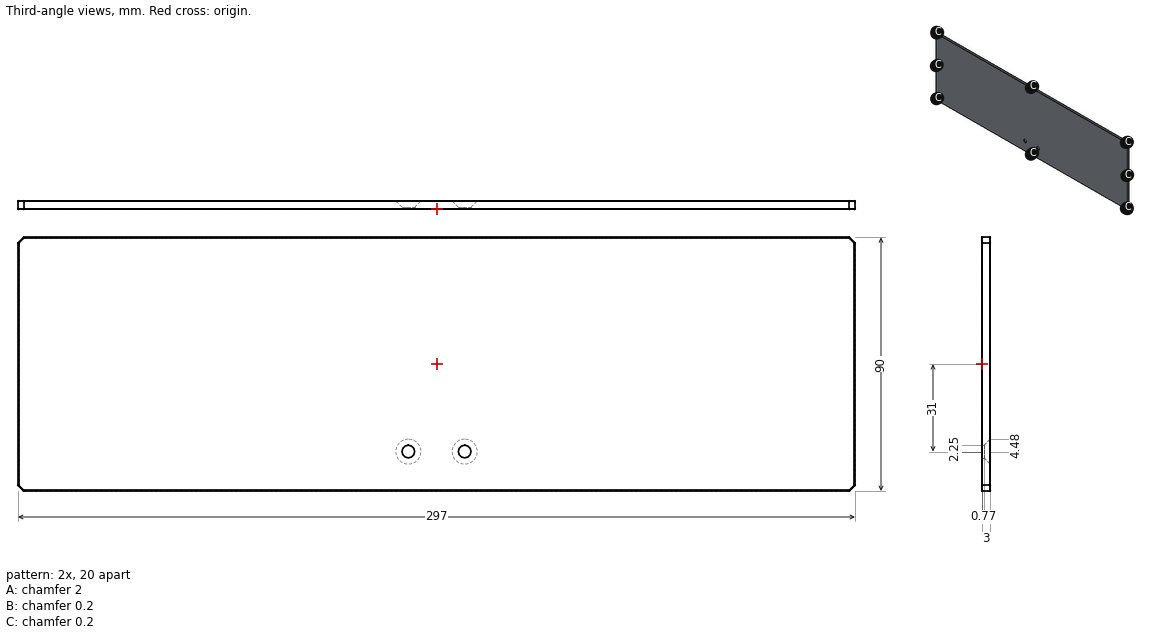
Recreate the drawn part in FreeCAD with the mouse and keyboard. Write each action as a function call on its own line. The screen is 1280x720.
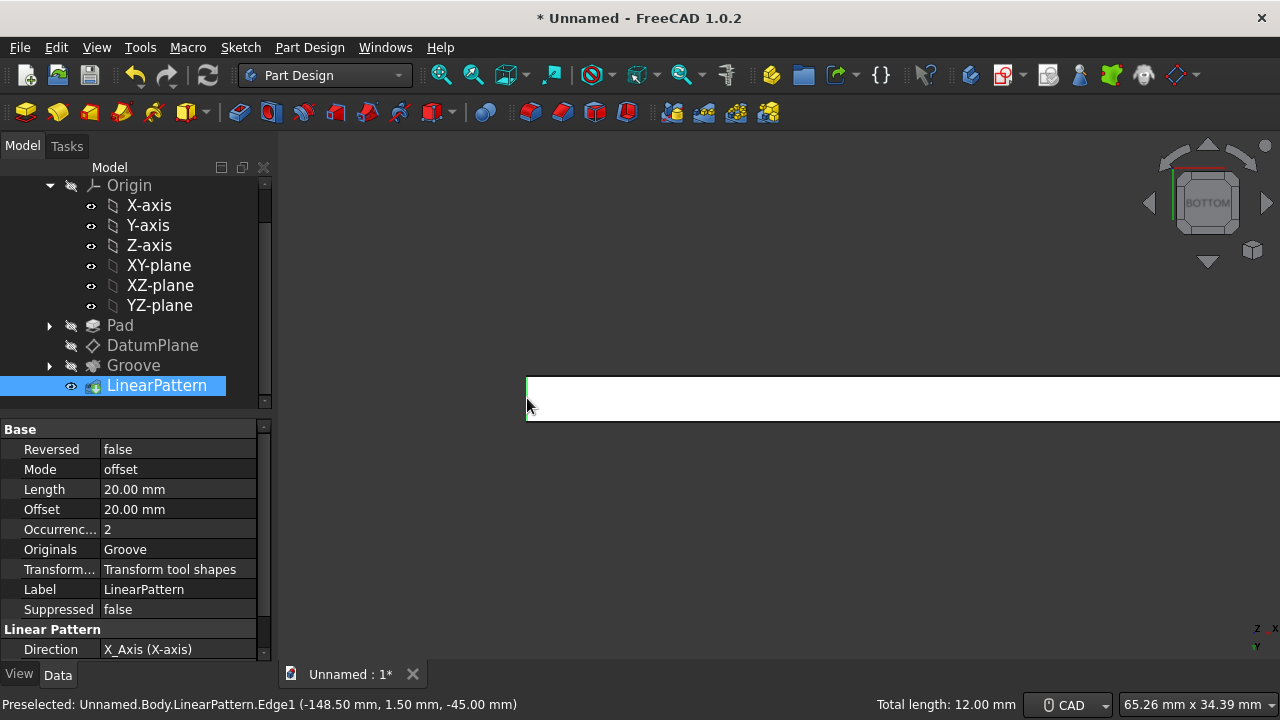
click(564, 112)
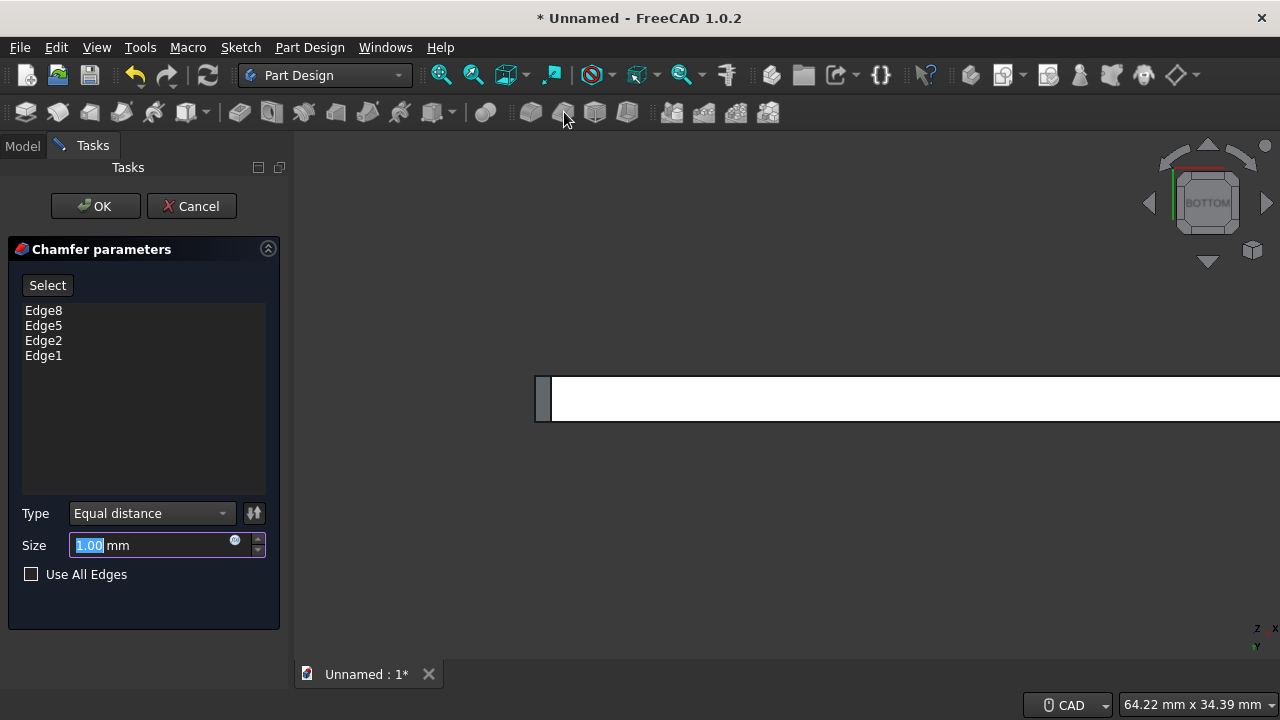
text(2)
key(Tab)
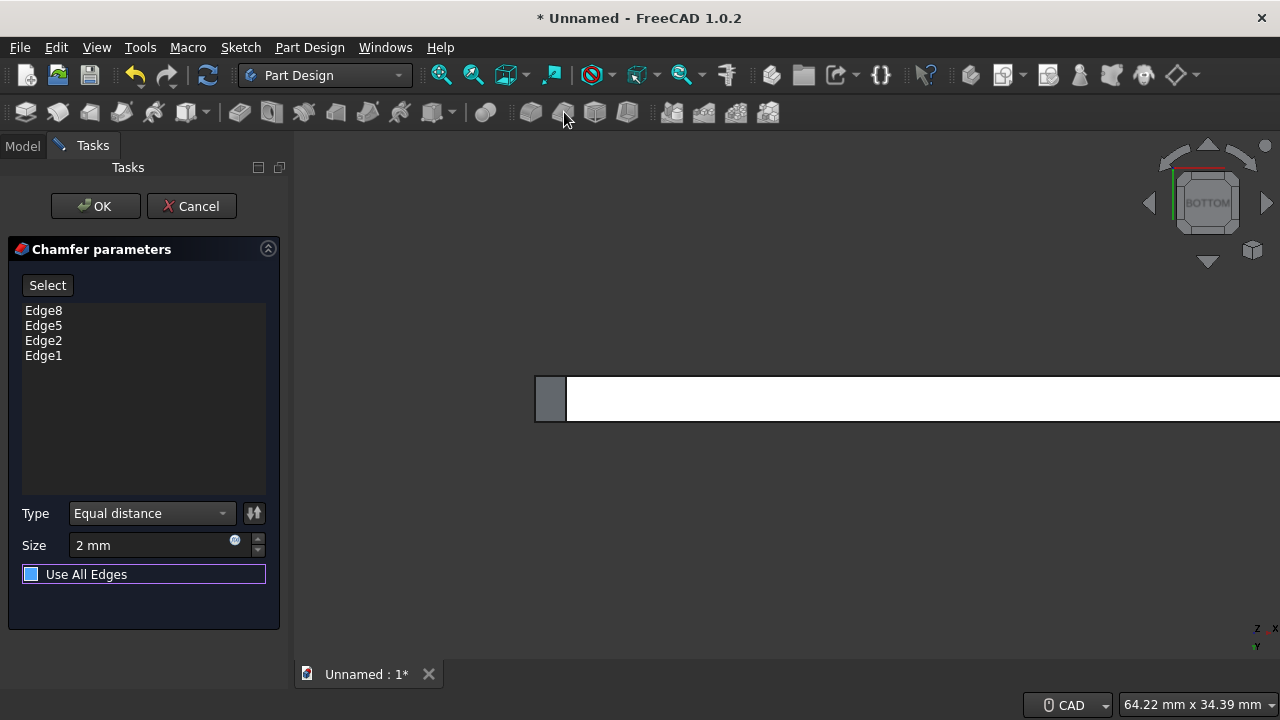
click(96, 206)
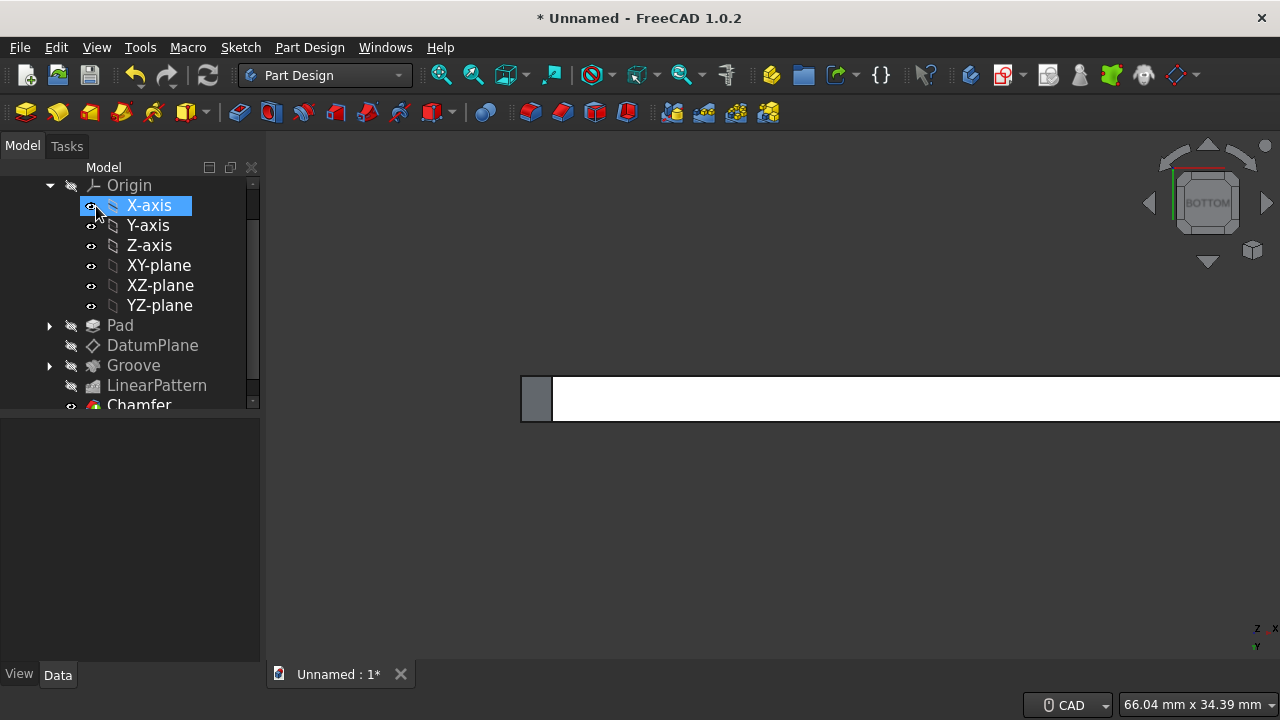
click(442, 76)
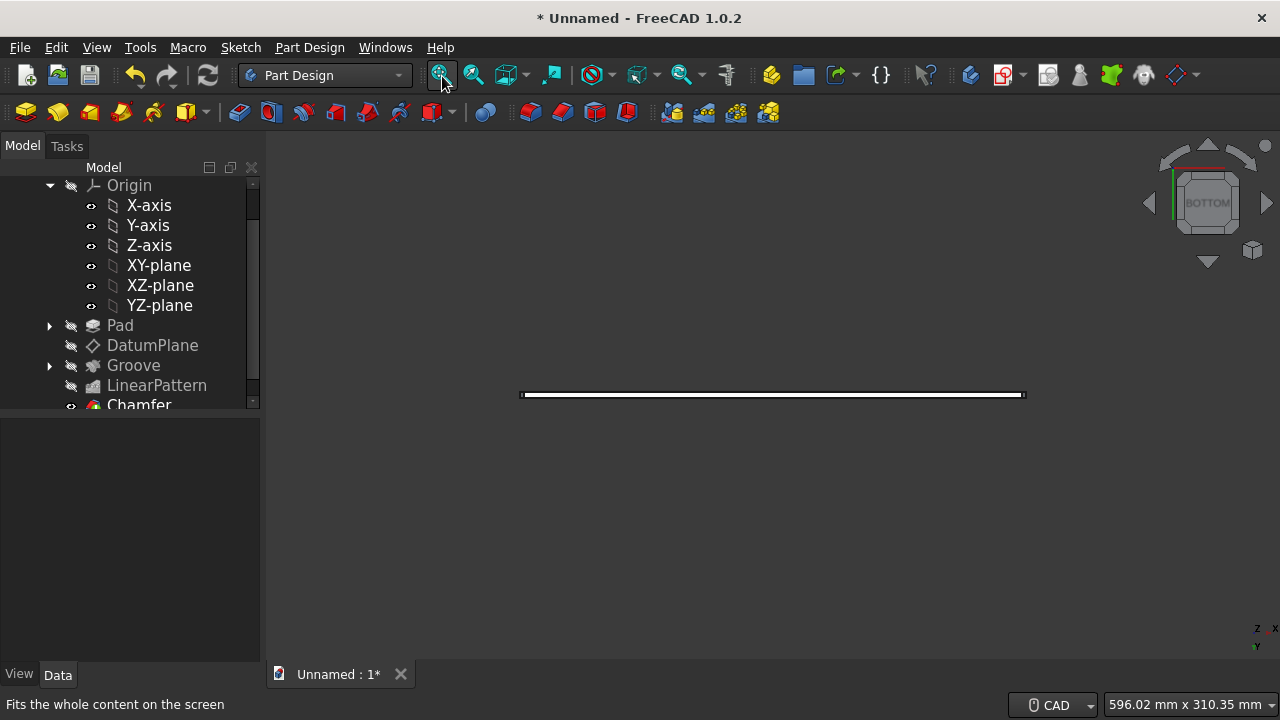
click(773, 391)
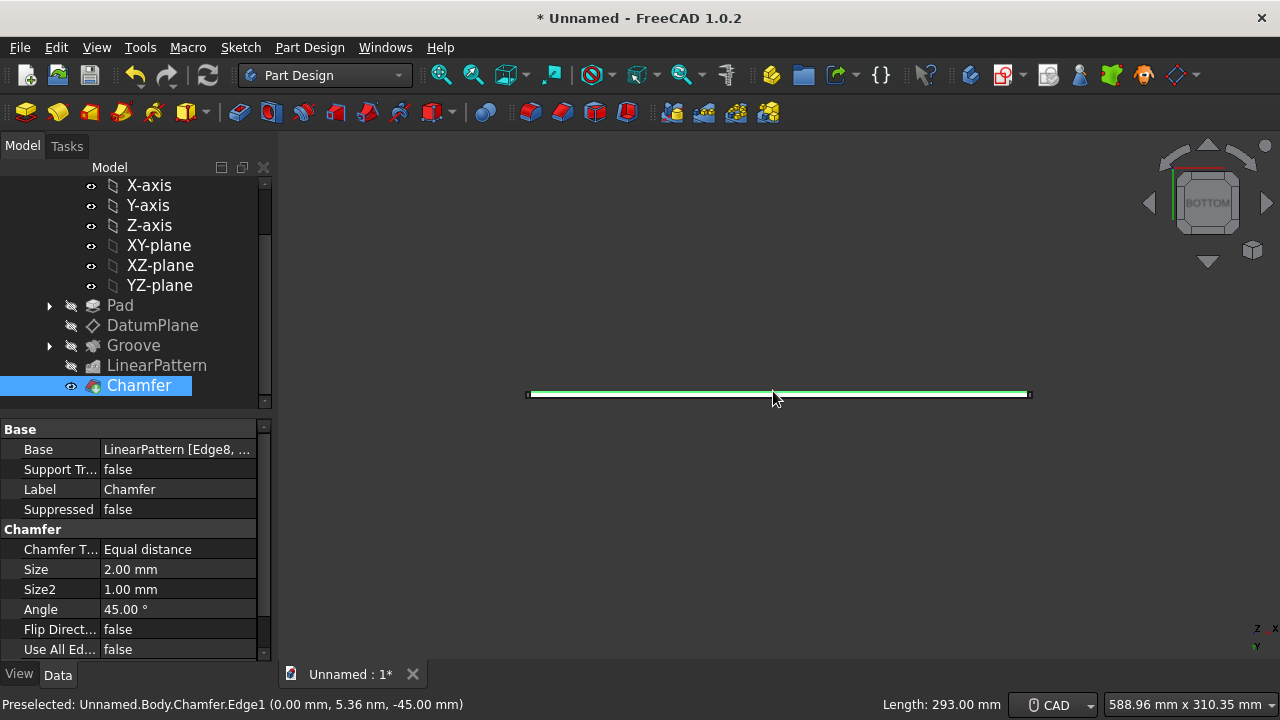
key(0)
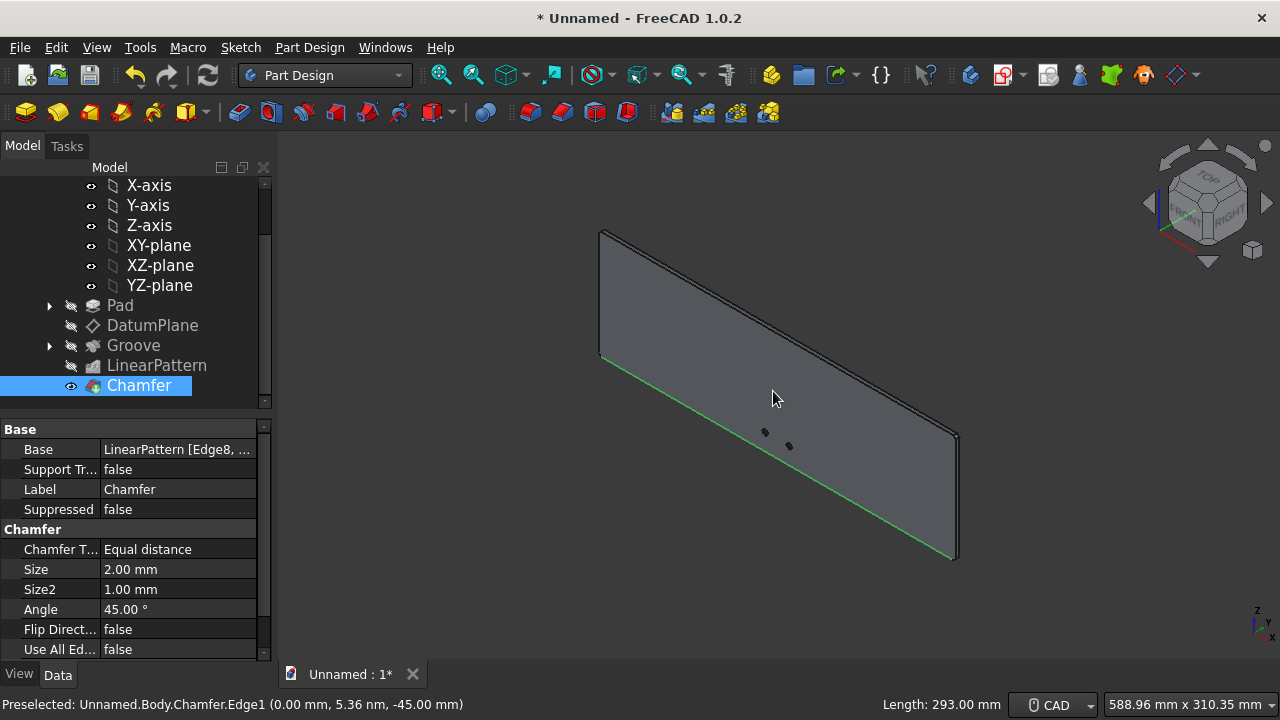
click(956, 498, ctrl)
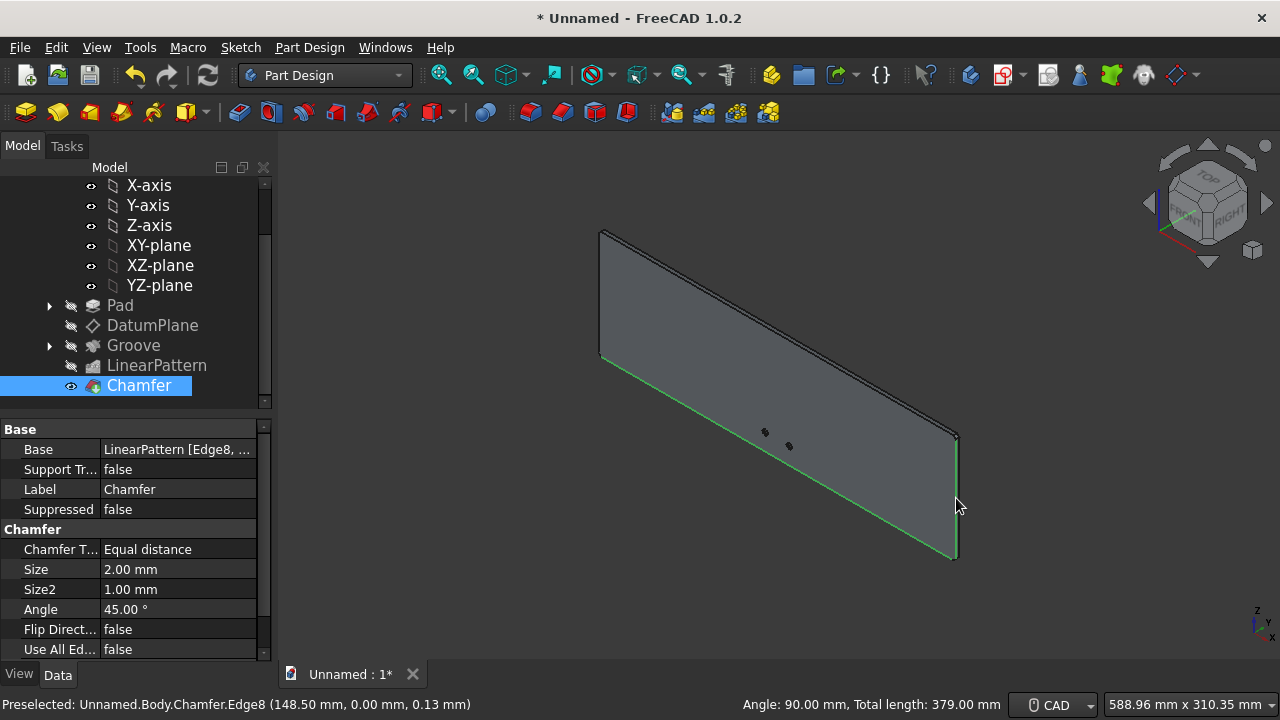
click(777, 333, ctrl)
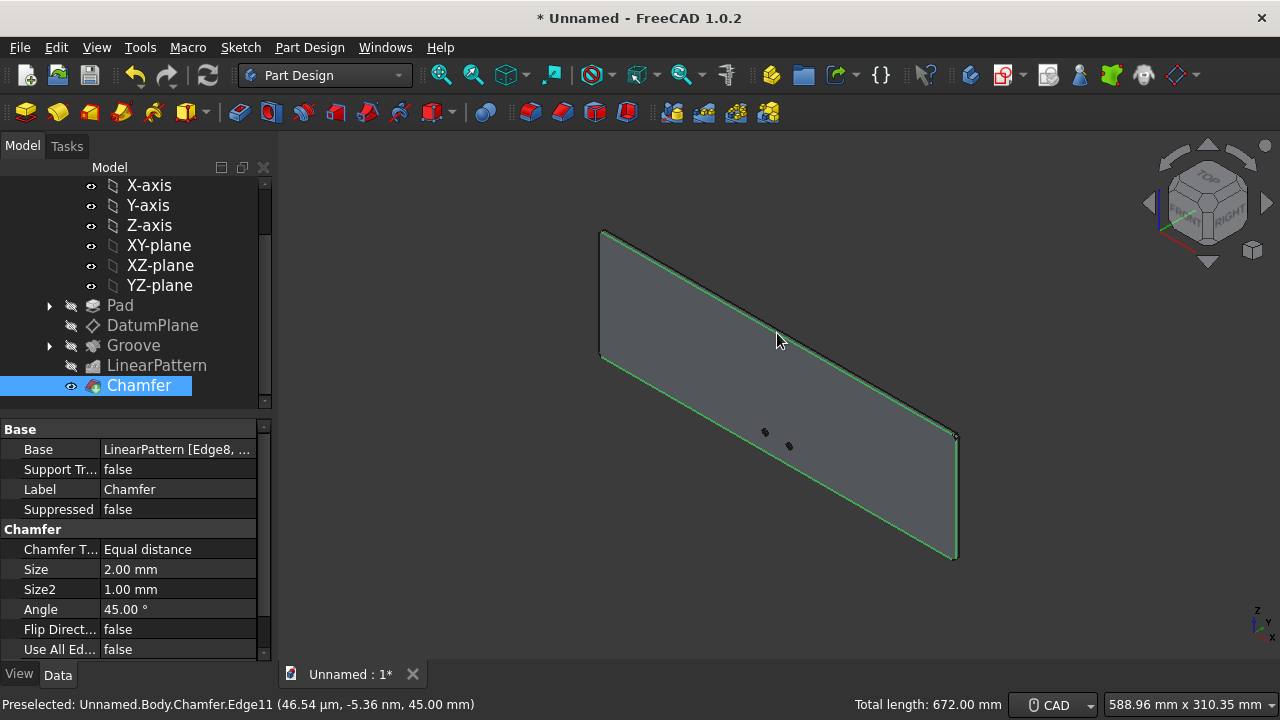
key(2)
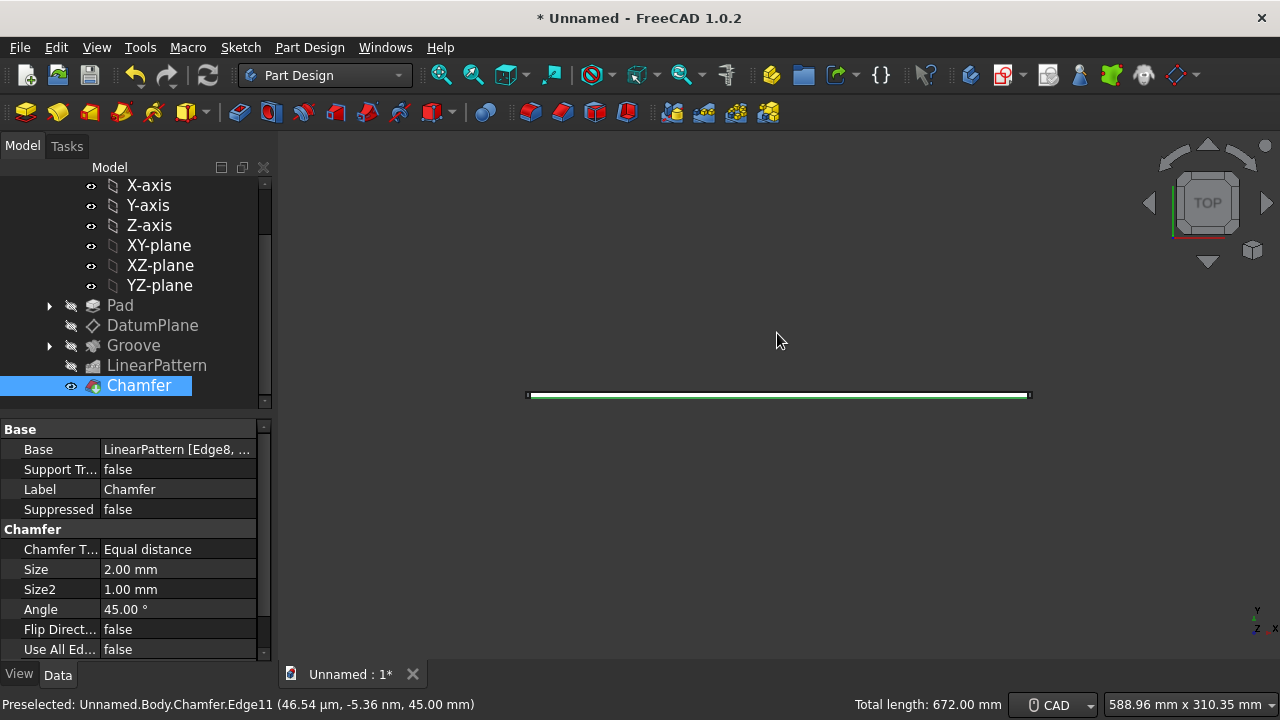
key(1)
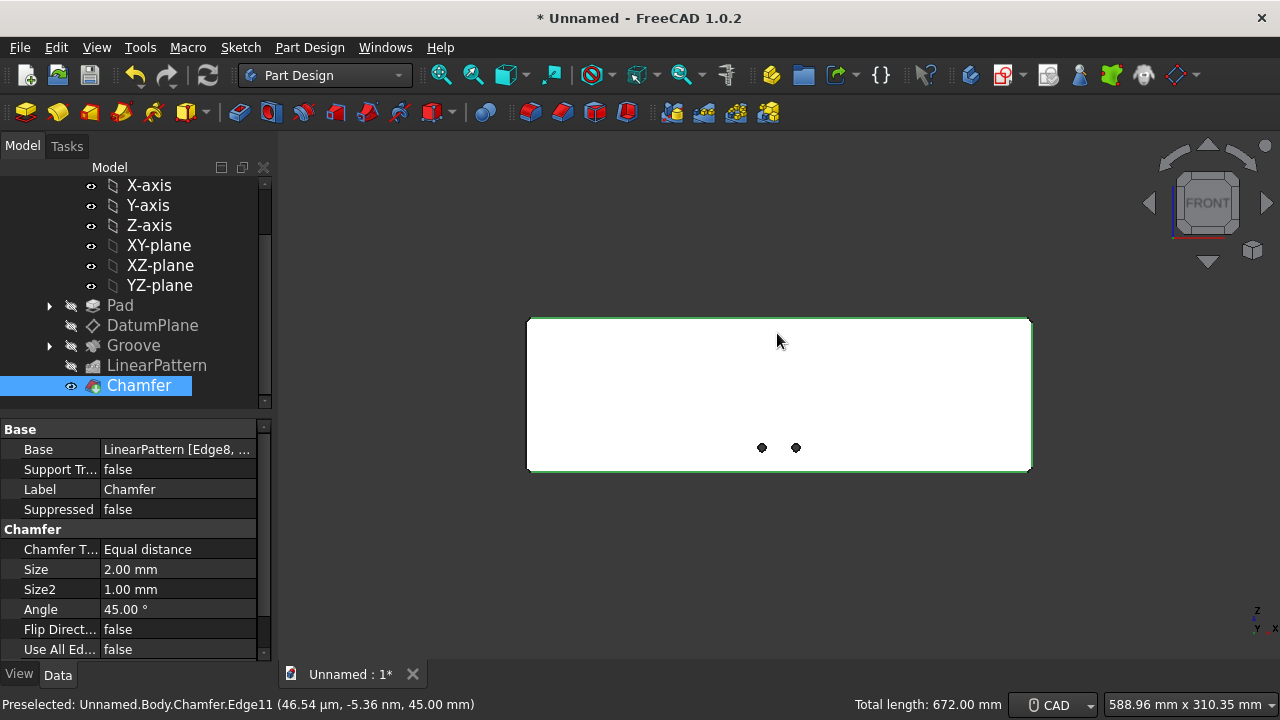
click(526, 379, ctrl)